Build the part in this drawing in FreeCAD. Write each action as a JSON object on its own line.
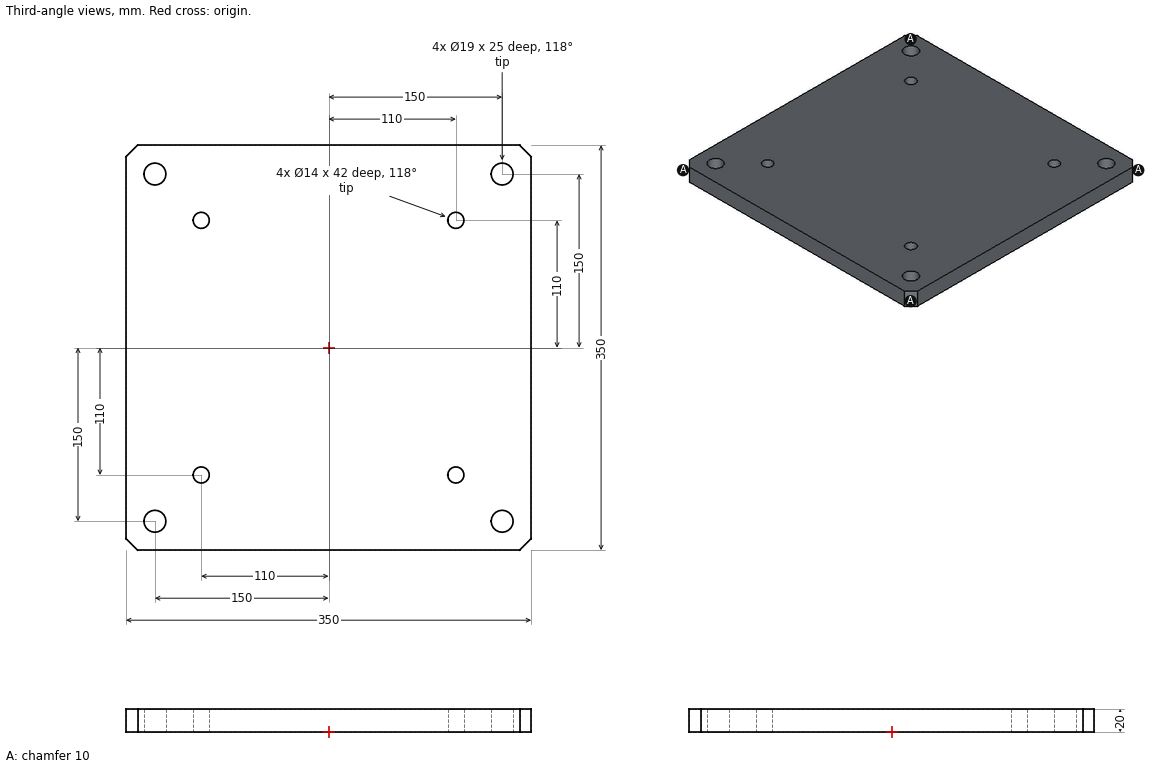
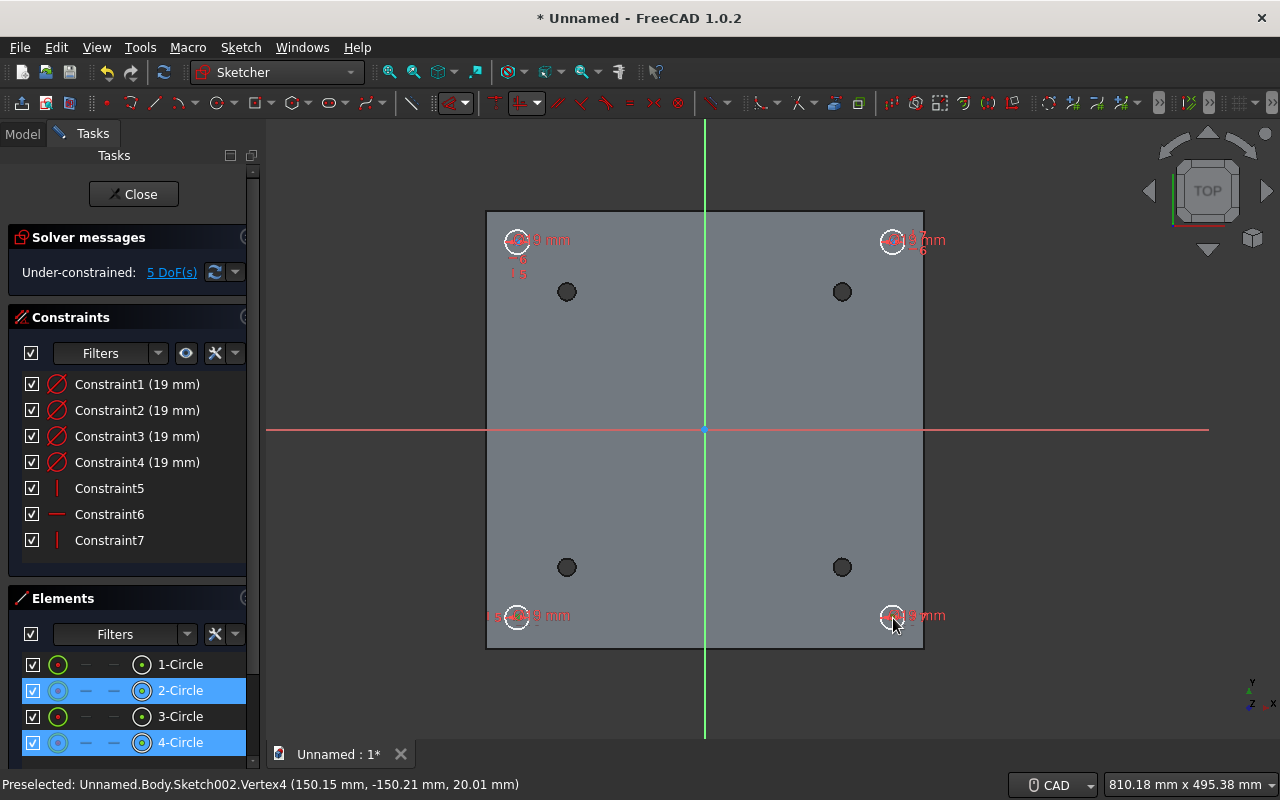
{"action": "left_click", "coordinate": [540, 104]}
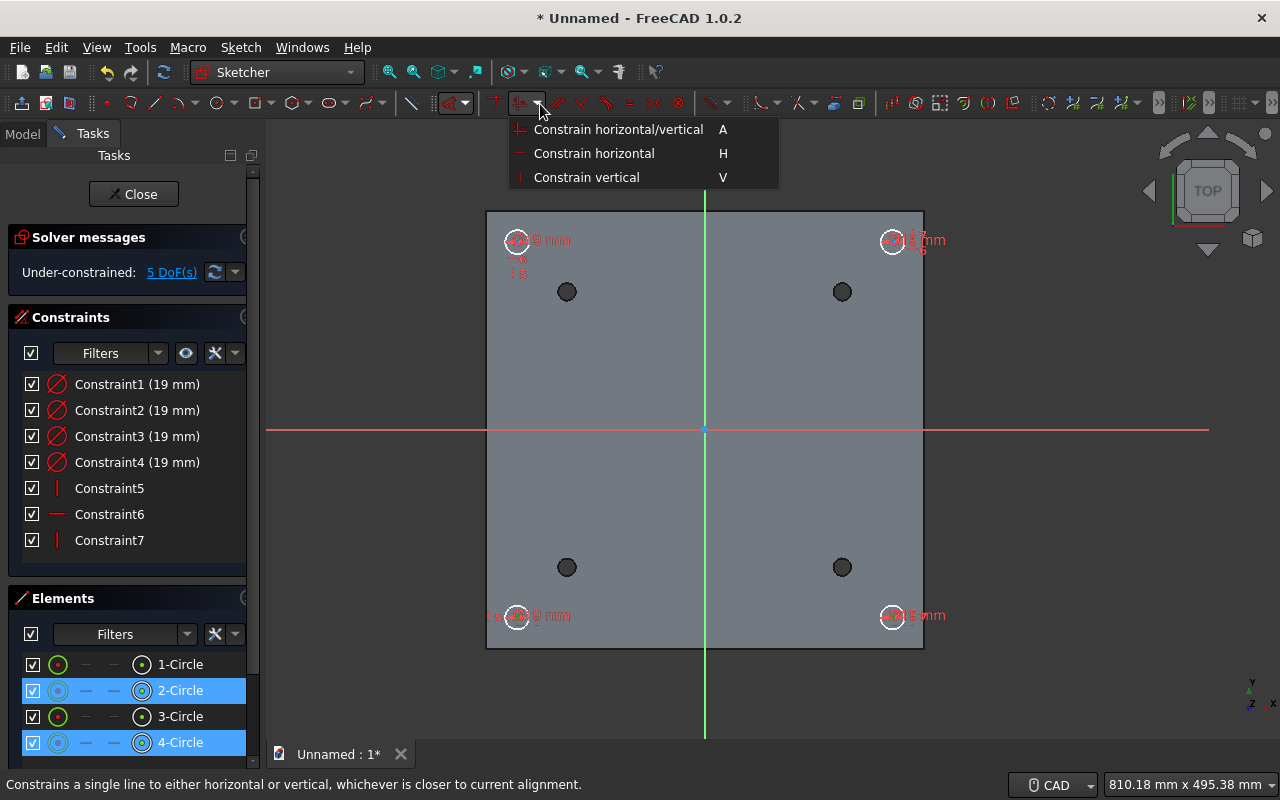
{"action": "left_click", "coordinate": [644, 153]}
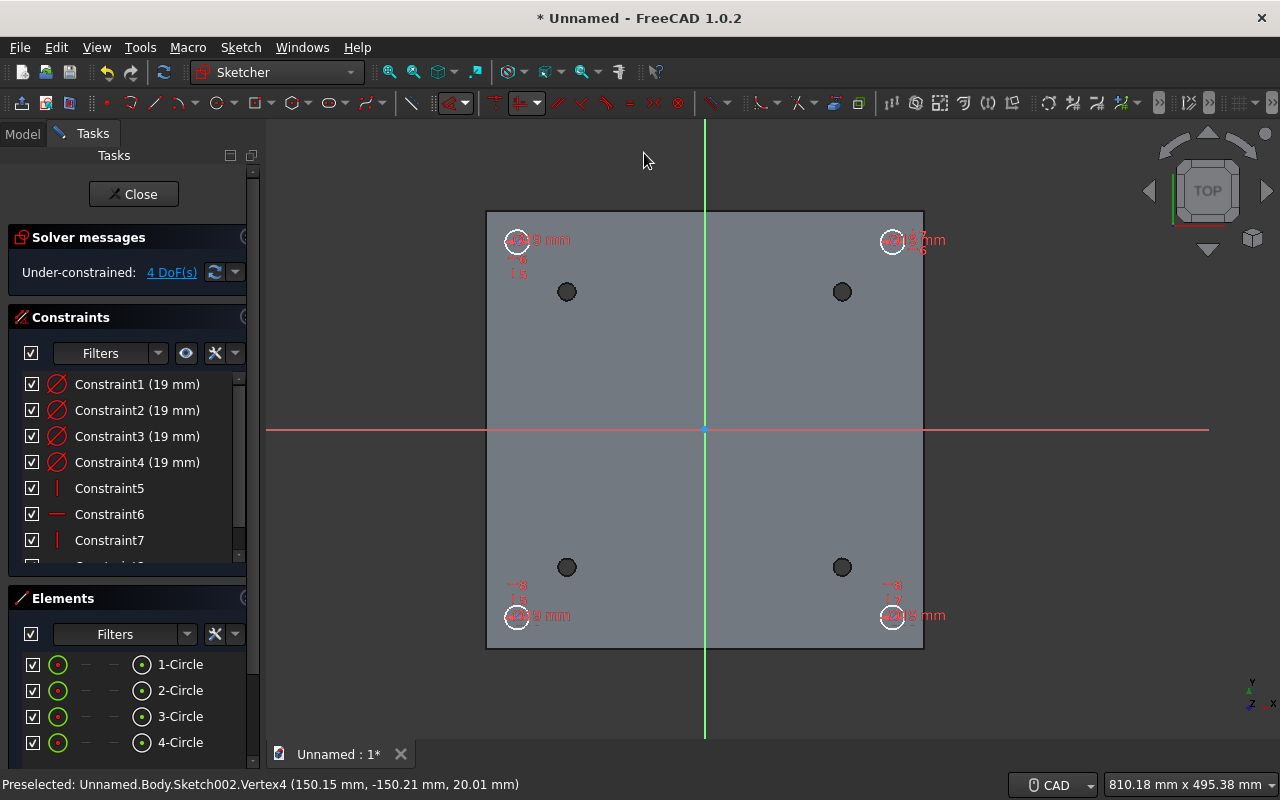
{"action": "left_click", "coordinate": [893, 242]}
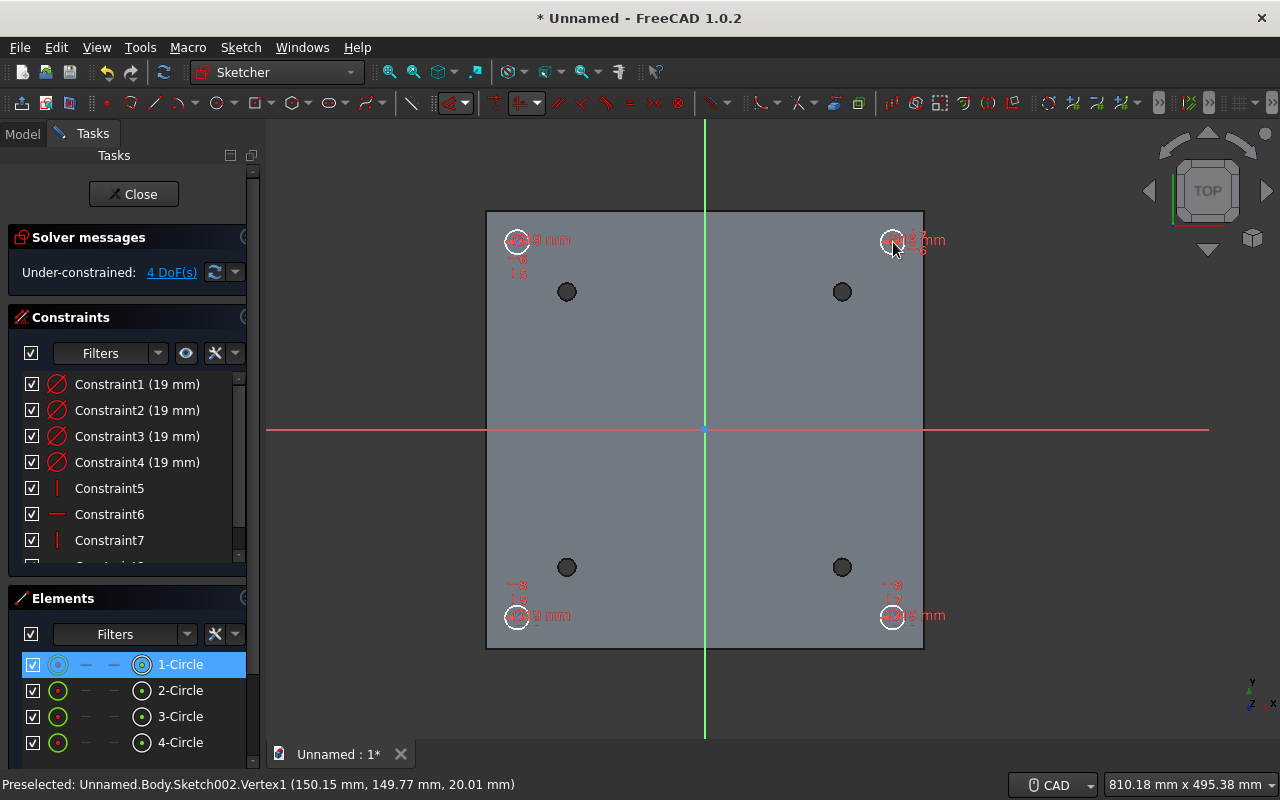
{"action": "key", "text": "l"}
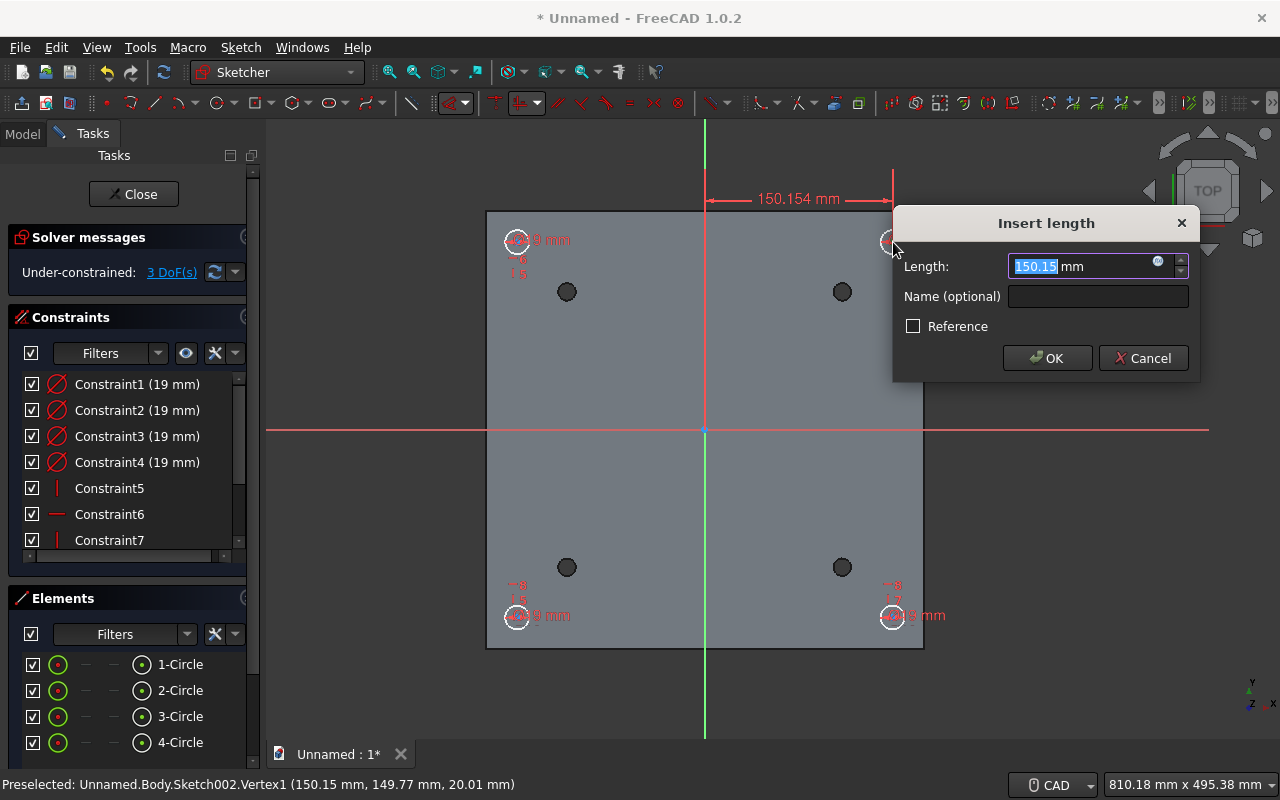
{"action": "type", "text": "150"}
{"action": "key", "text": "Return"}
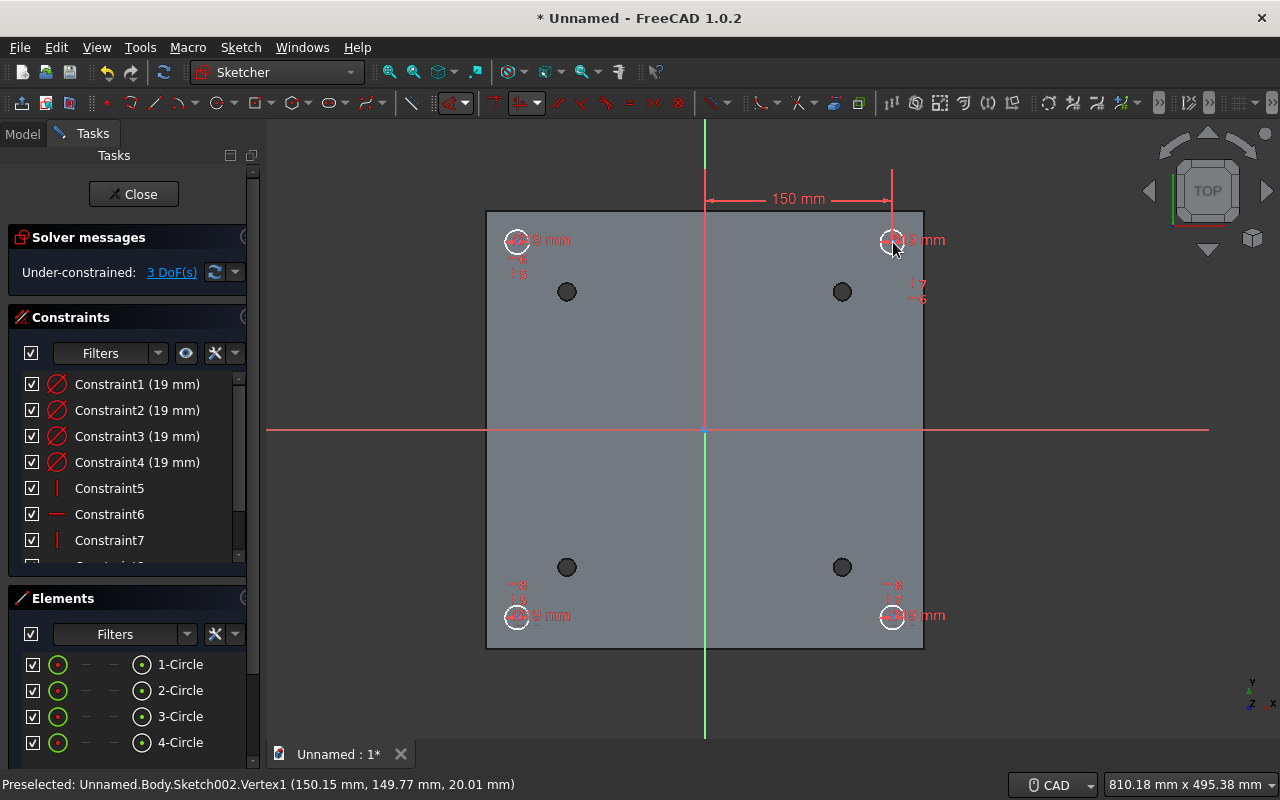
{"action": "left_click", "coordinate": [892, 242]}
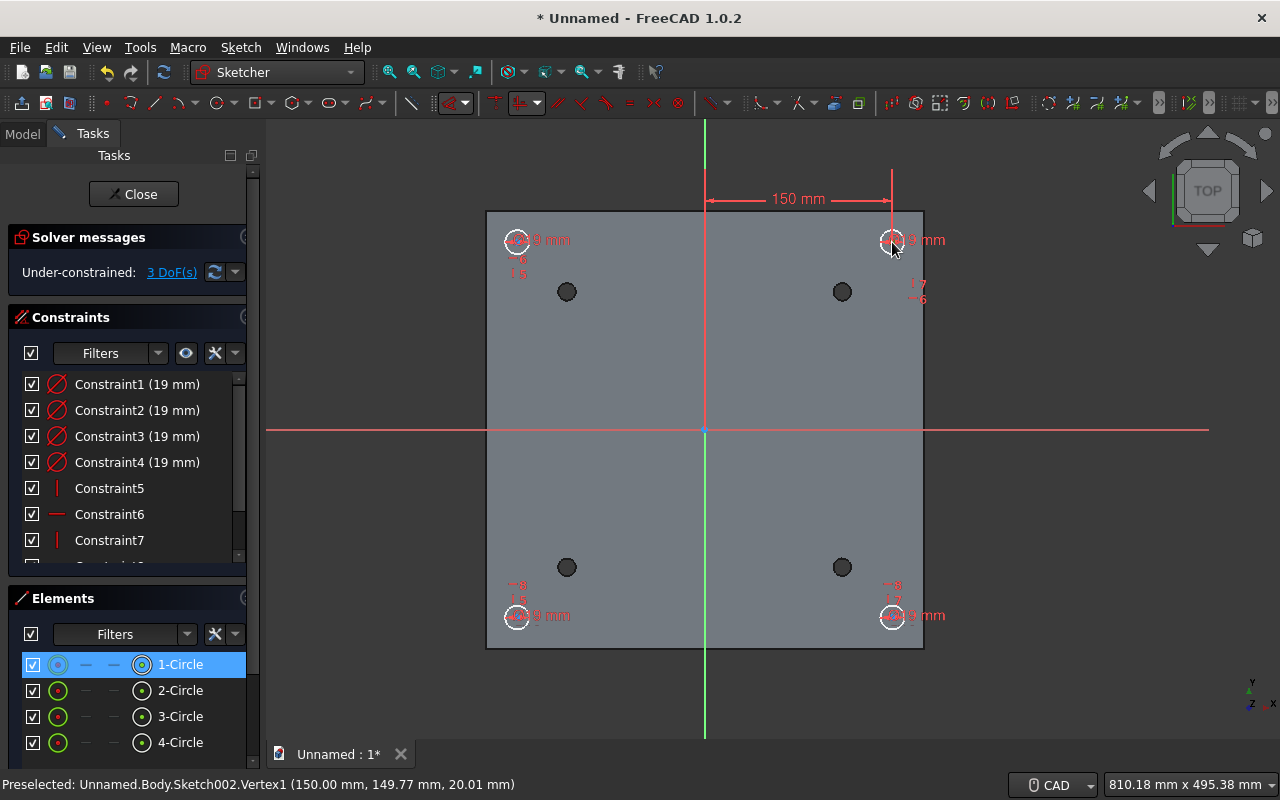
{"action": "left_click", "coordinate": [468, 104]}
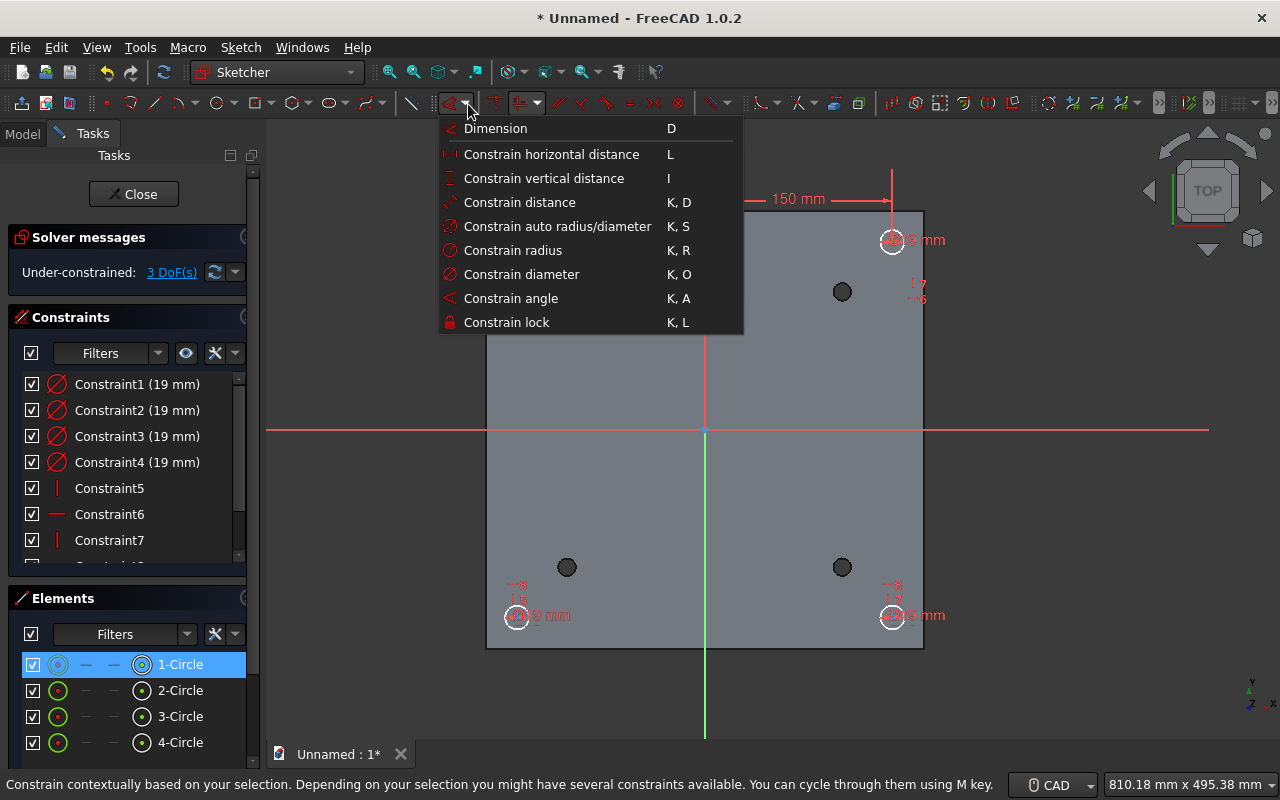
{"action": "left_click", "coordinate": [591, 178]}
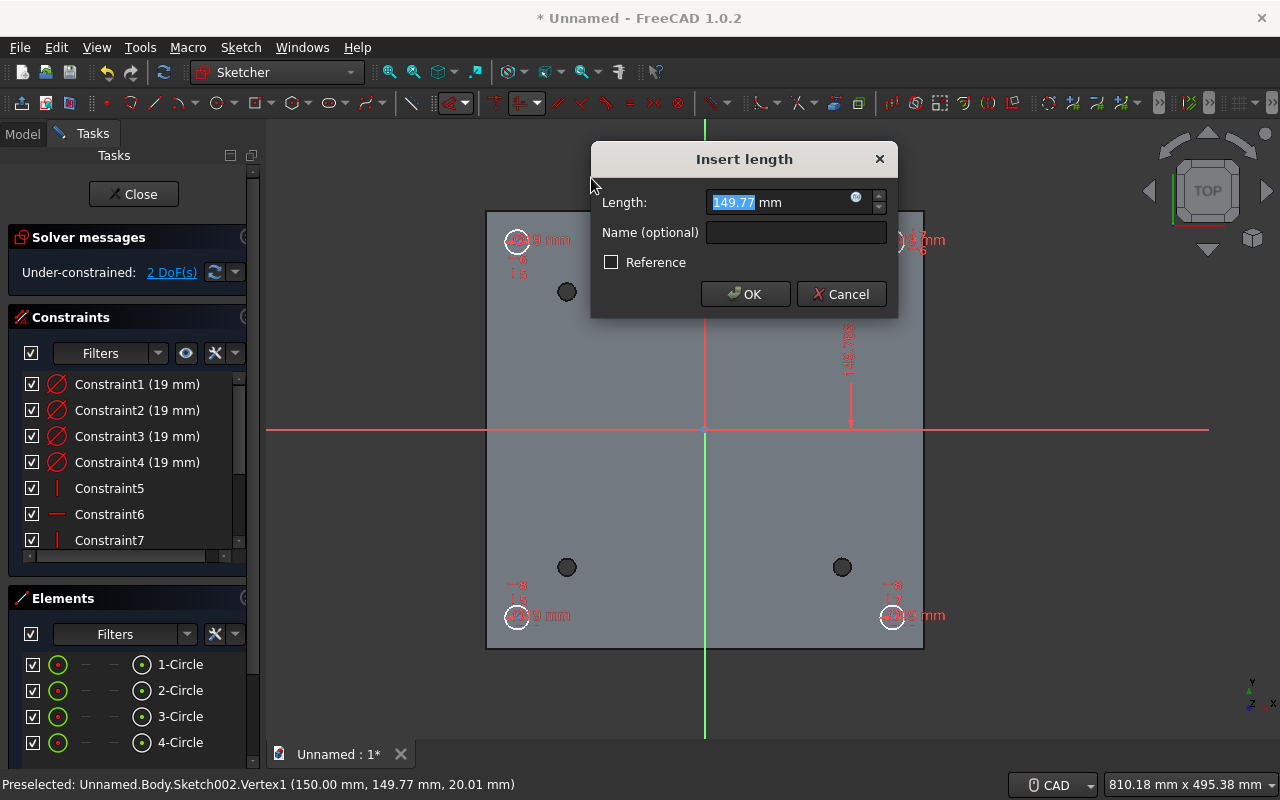
{"action": "type", "text": "150"}
{"action": "key", "text": "Return"}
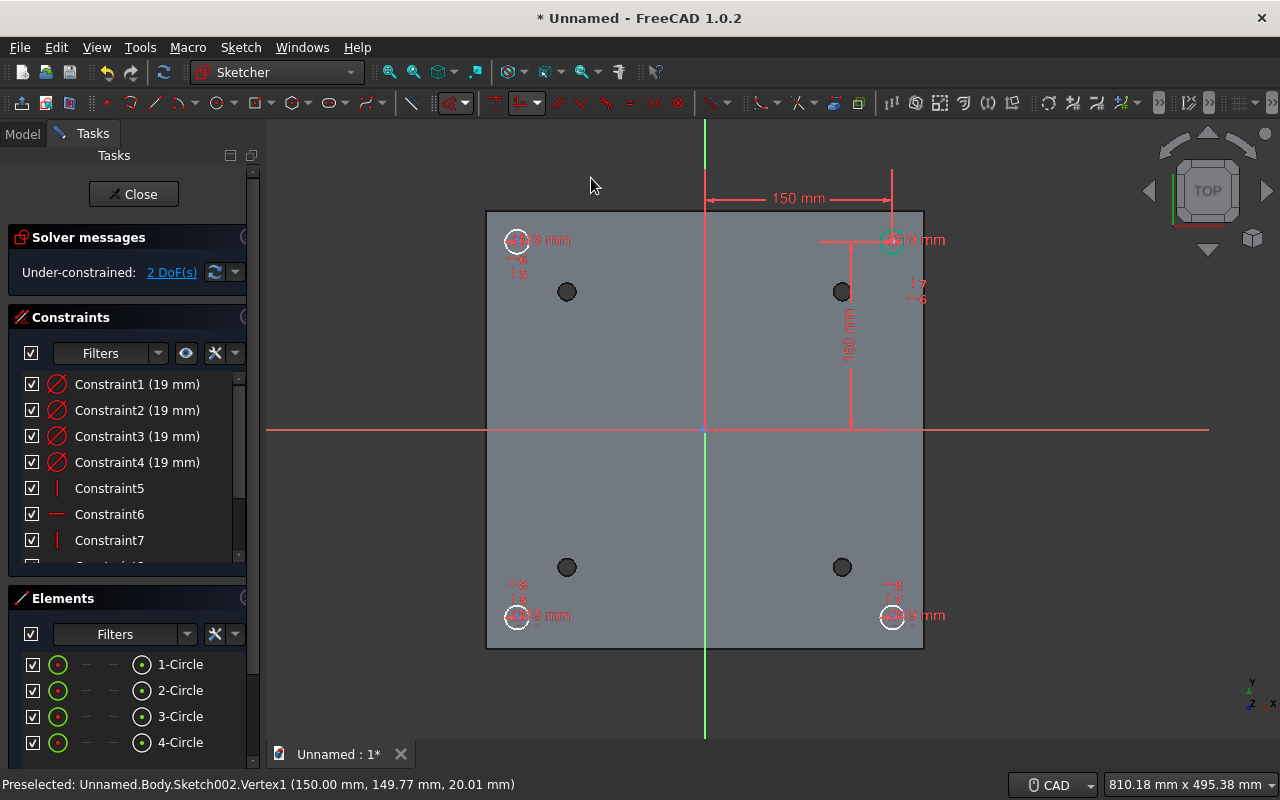
{"action": "left_click", "coordinate": [517, 618]}